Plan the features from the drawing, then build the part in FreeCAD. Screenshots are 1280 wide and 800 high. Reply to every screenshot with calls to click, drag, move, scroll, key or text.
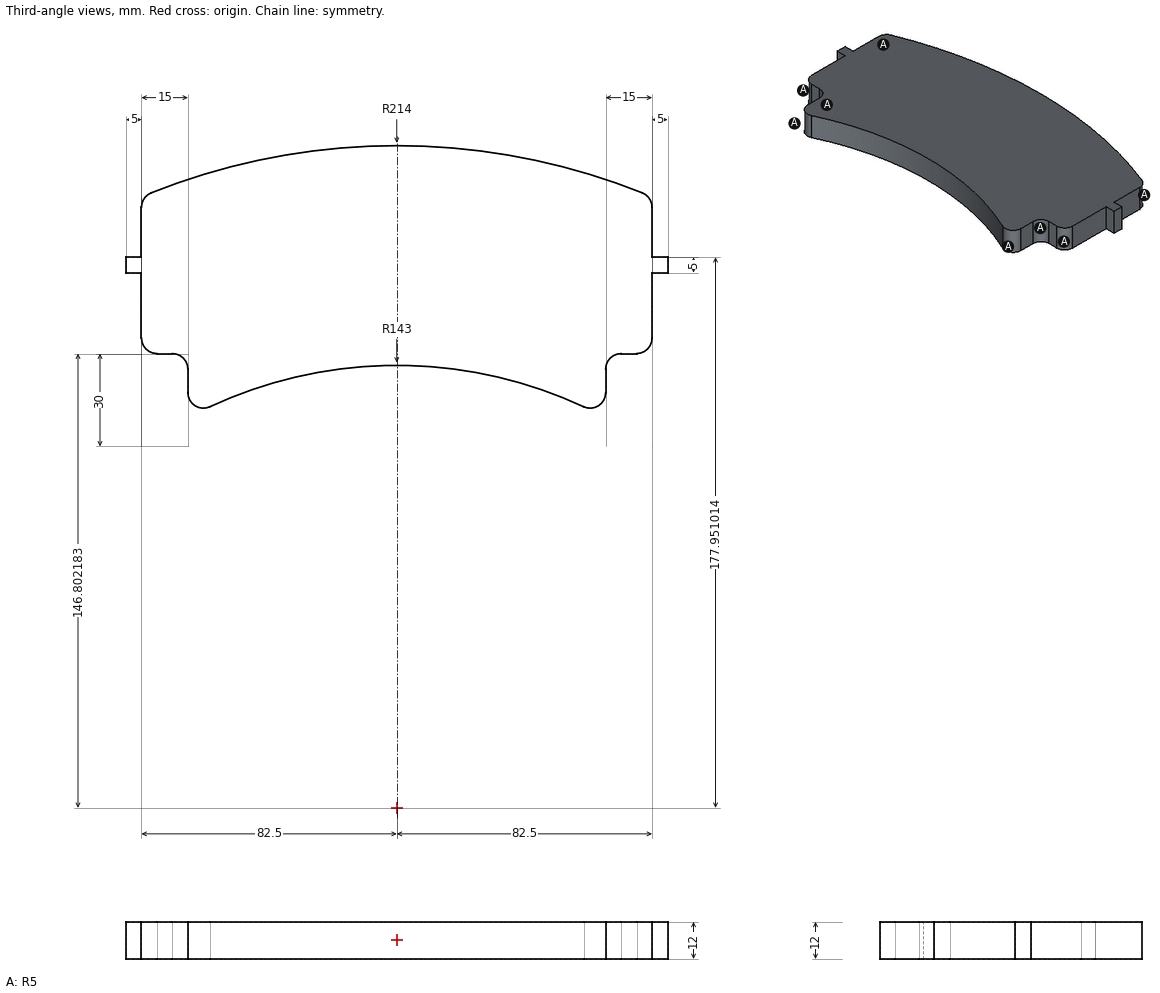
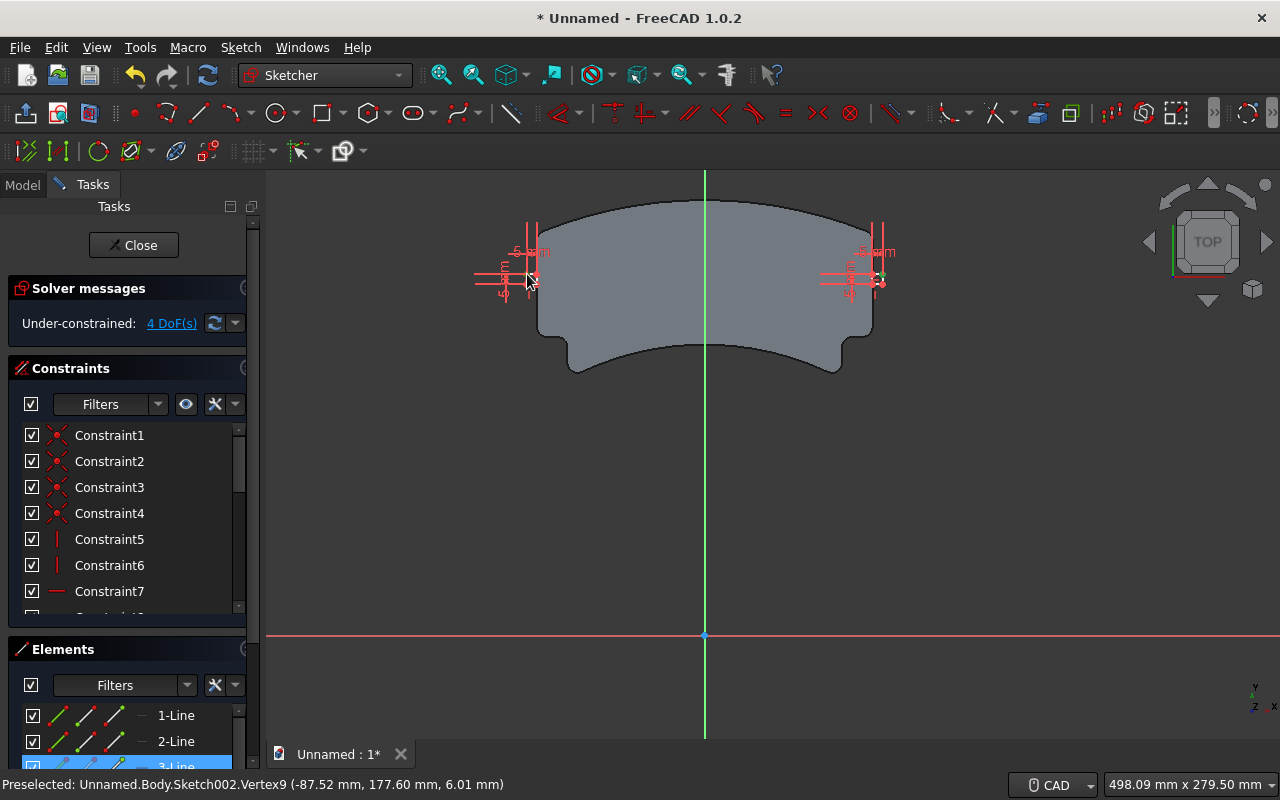
click(705, 674)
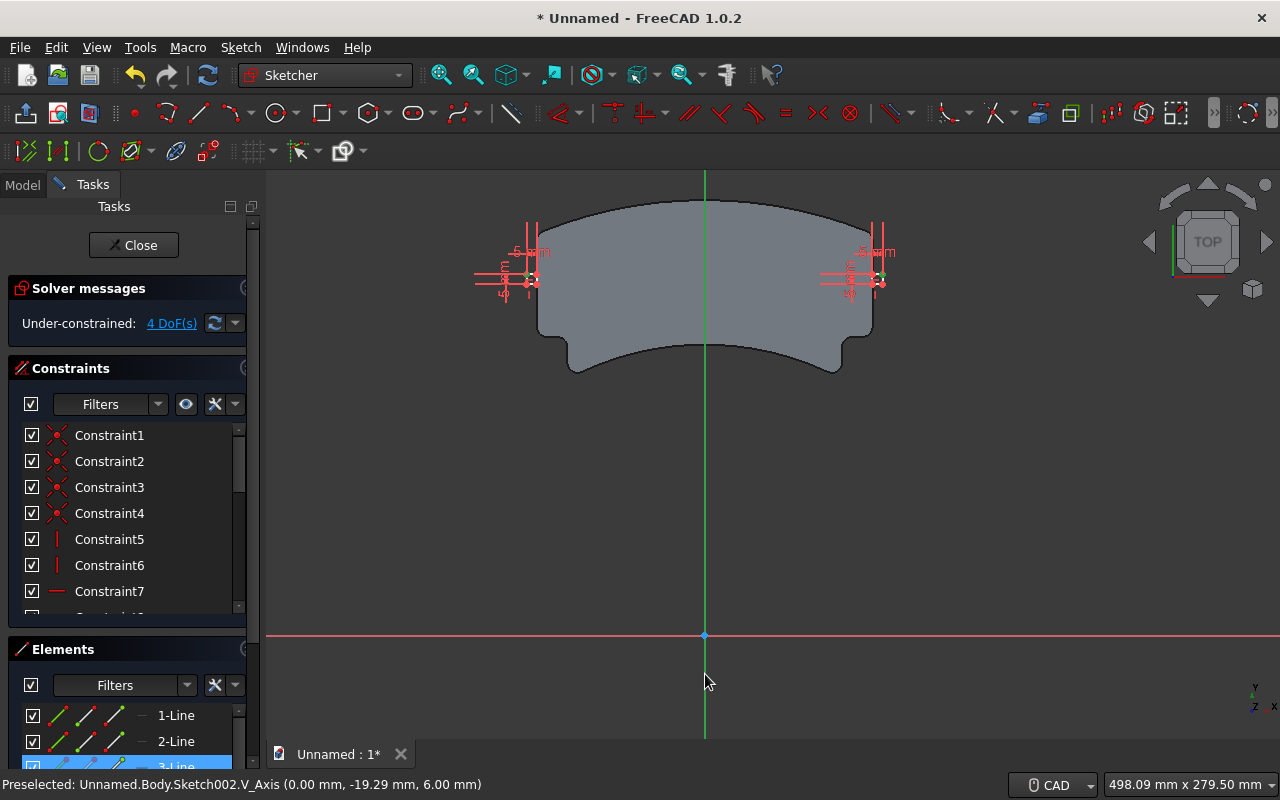
click(818, 114)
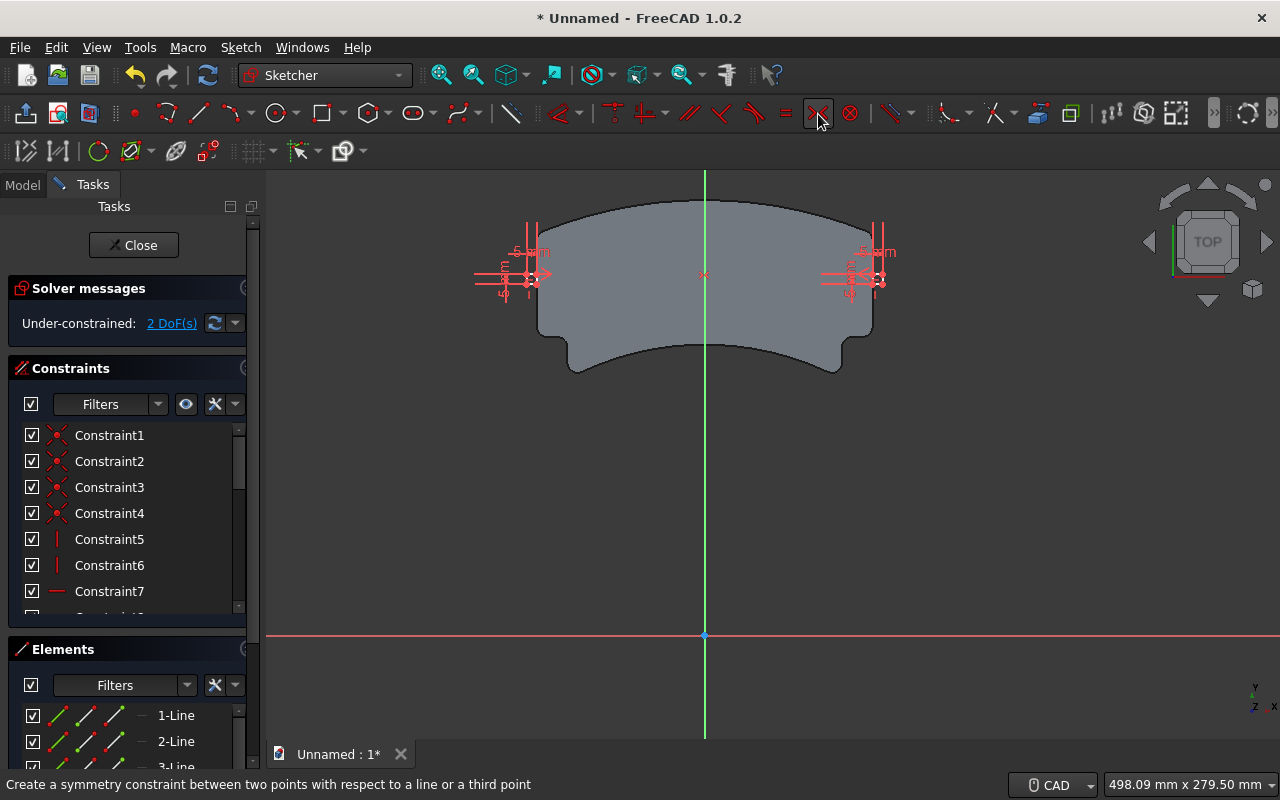
click(558, 114)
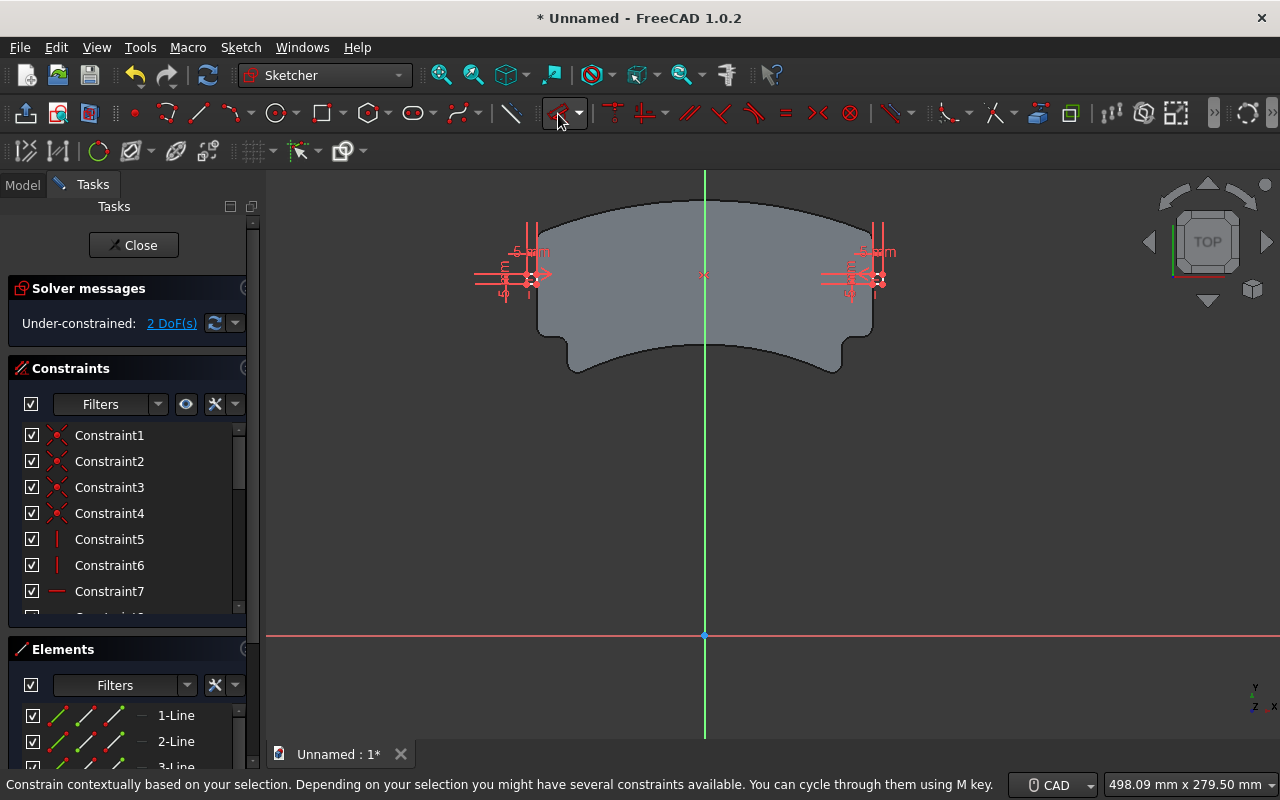
click(873, 274)
click(789, 670)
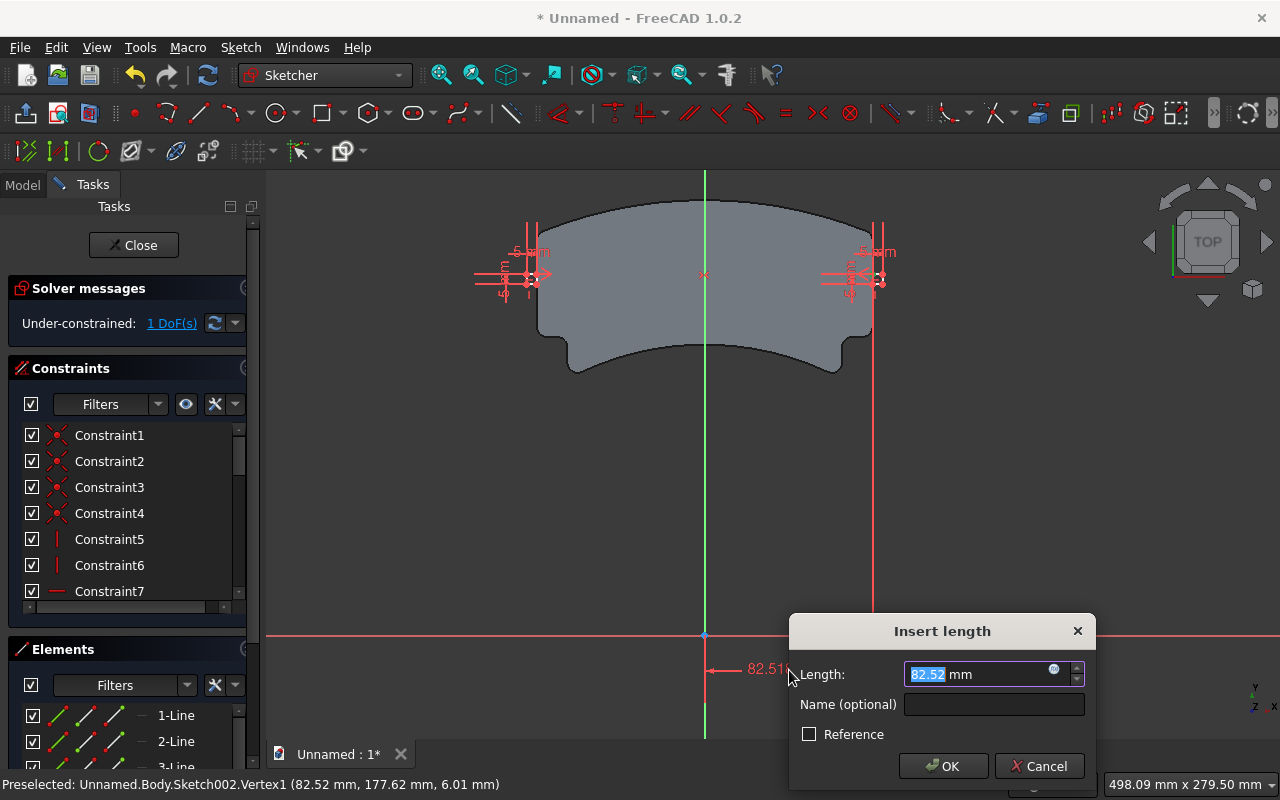
text(82.5)
key(Return)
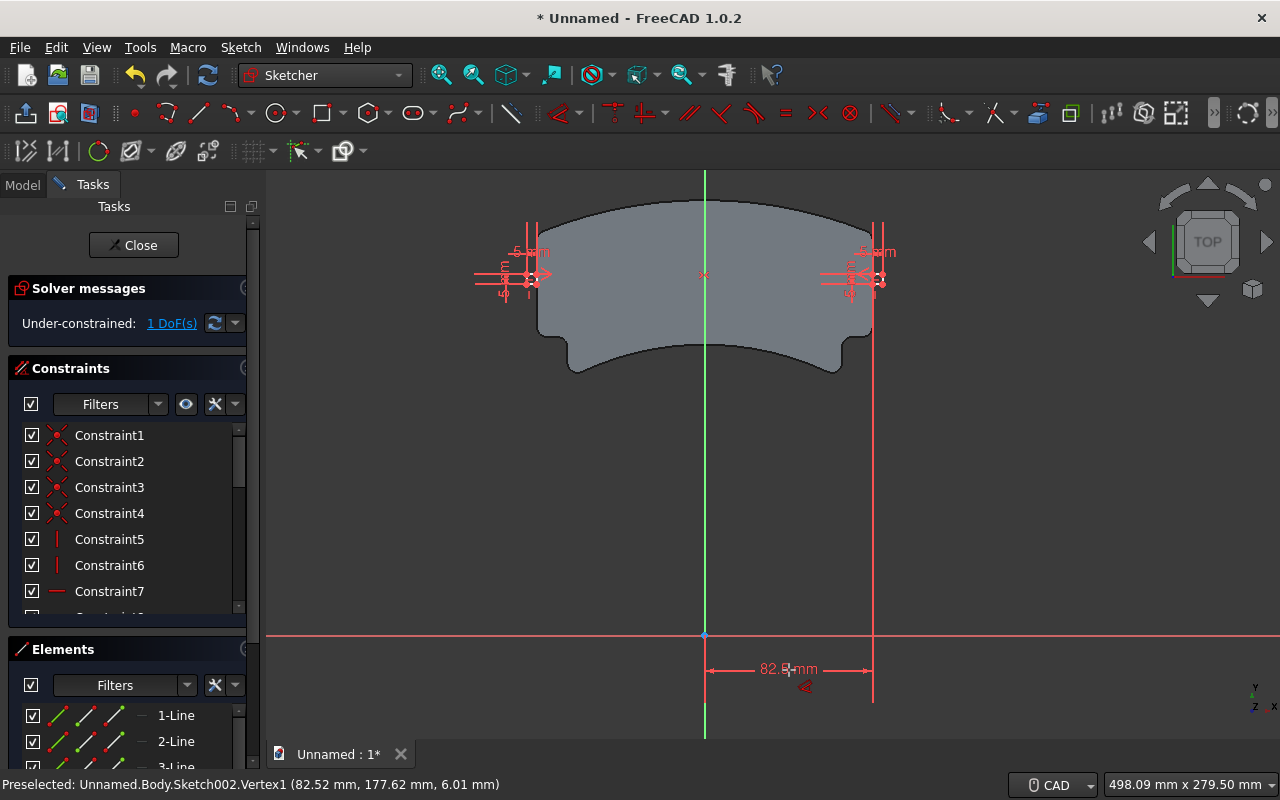
click(873, 274)
click(907, 455)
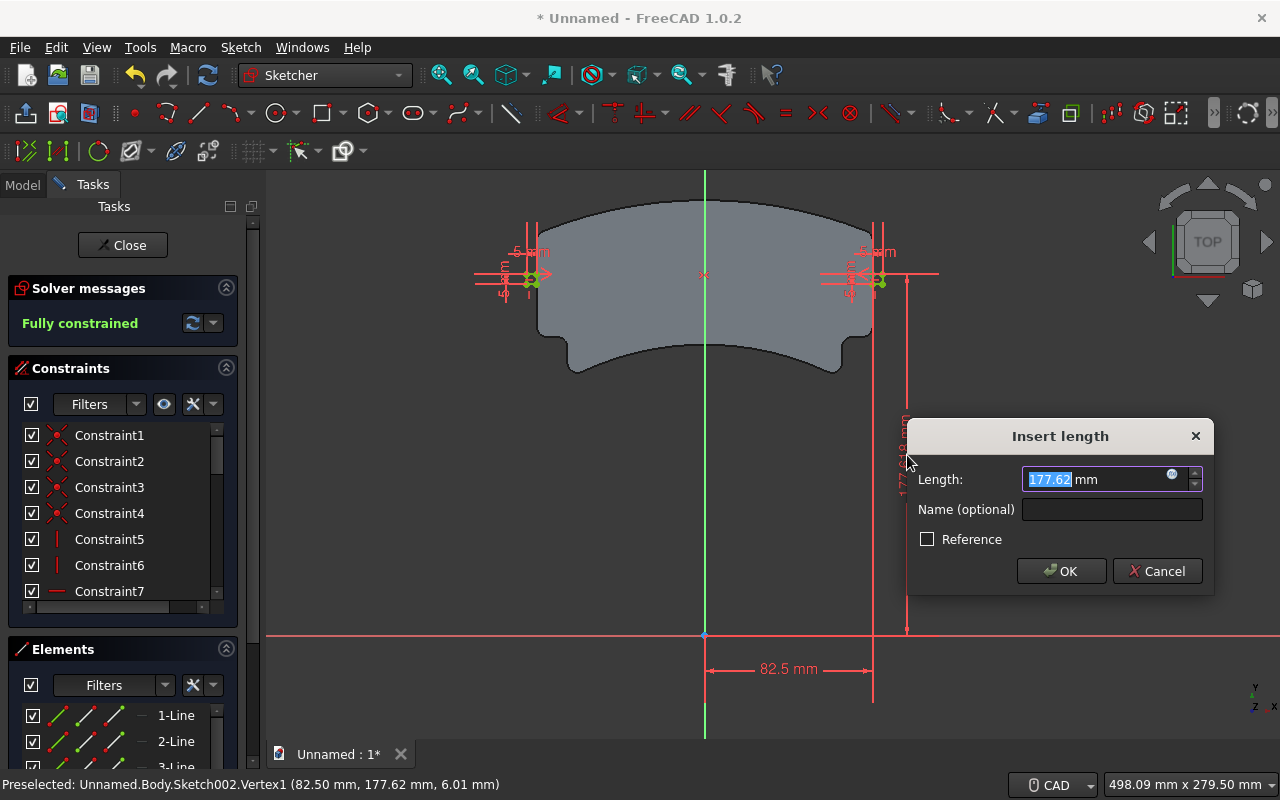
text(177.951014)
key(Return)
key(Escape)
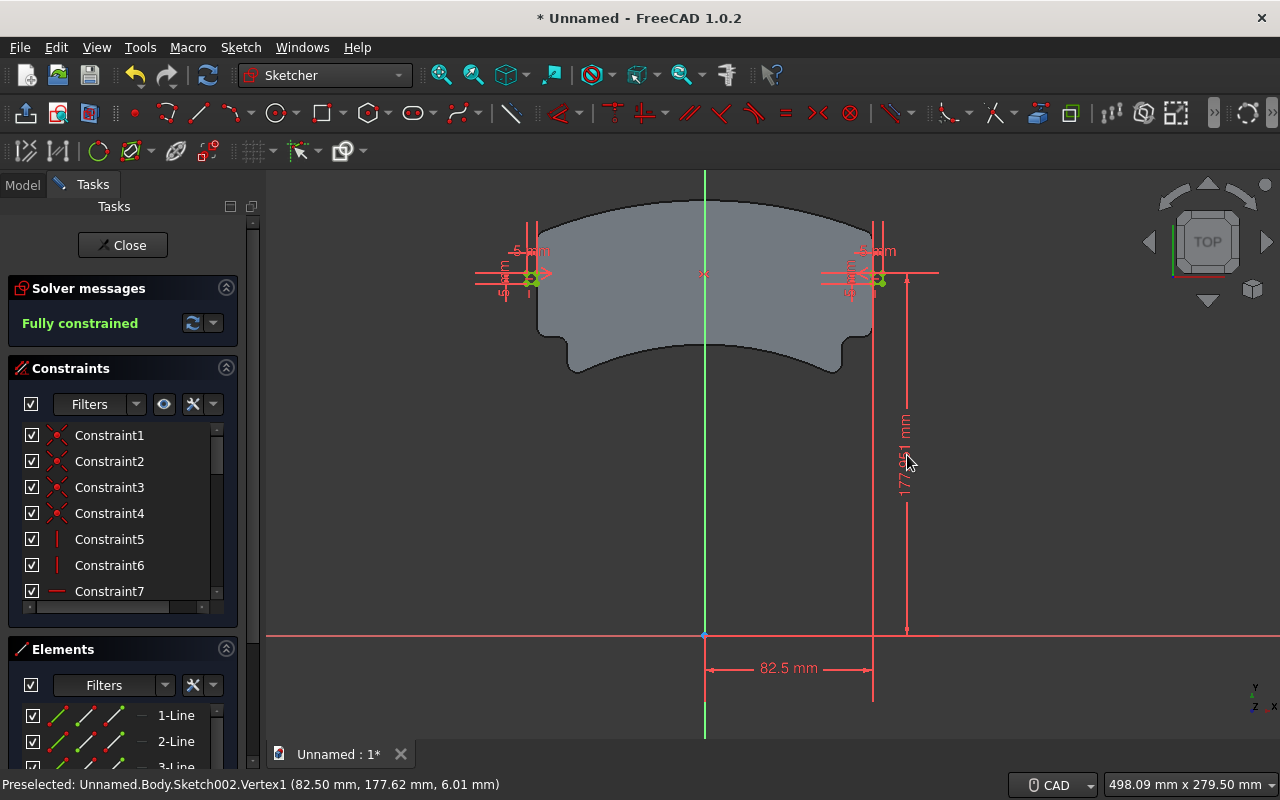
click(123, 245)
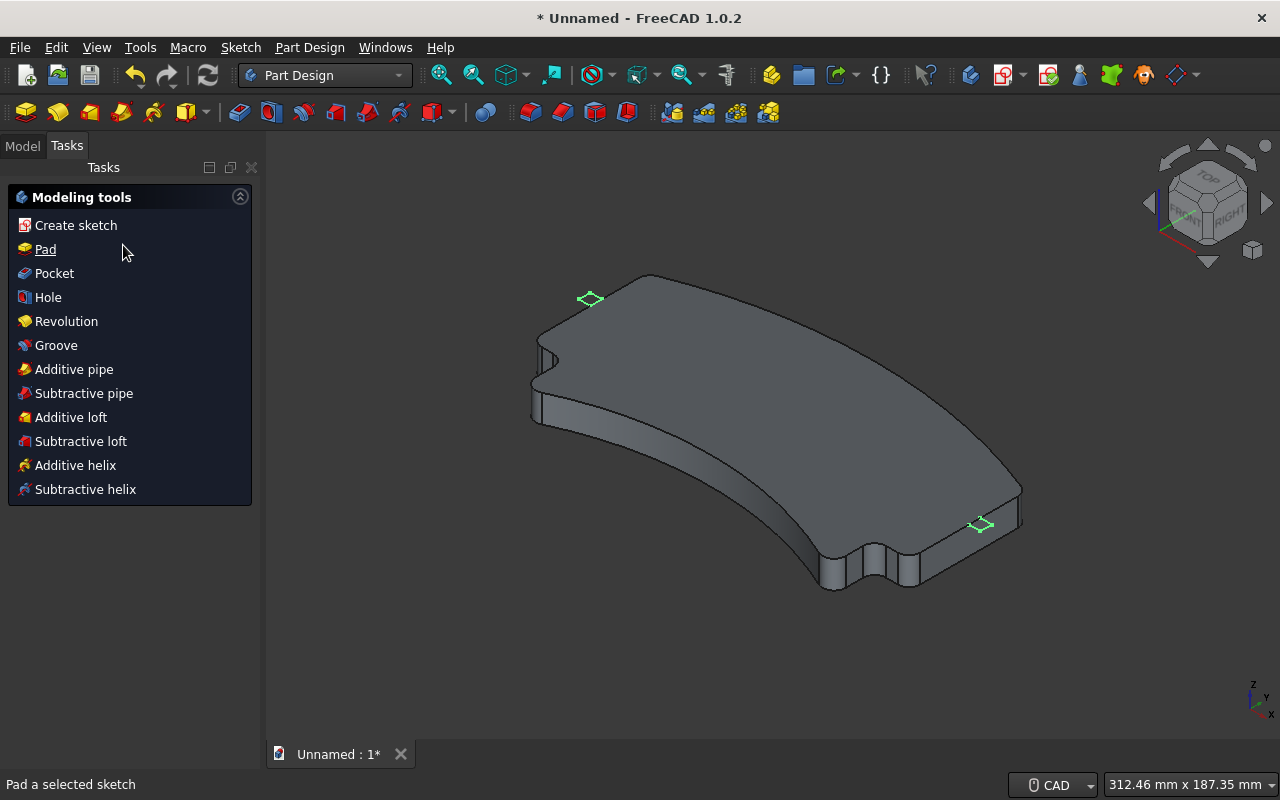
click(26, 112)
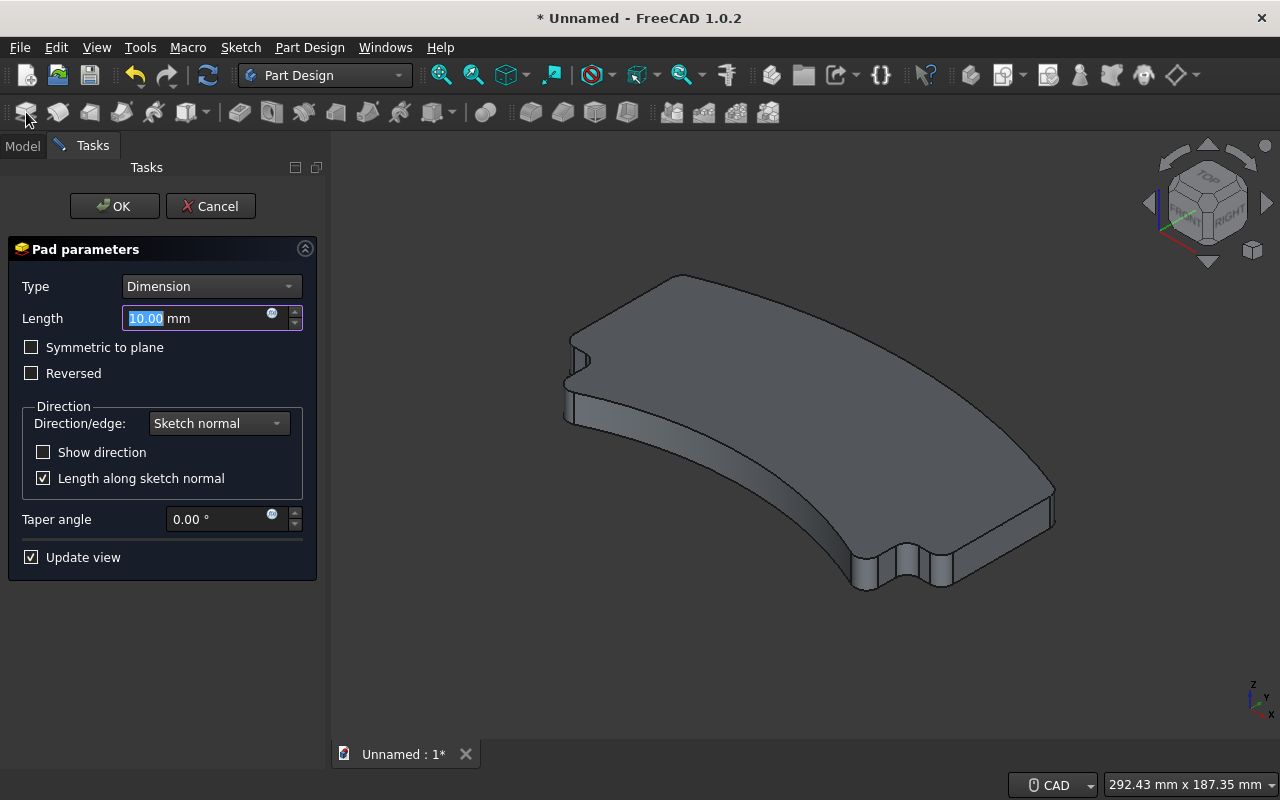
text(12)
key(Tab)